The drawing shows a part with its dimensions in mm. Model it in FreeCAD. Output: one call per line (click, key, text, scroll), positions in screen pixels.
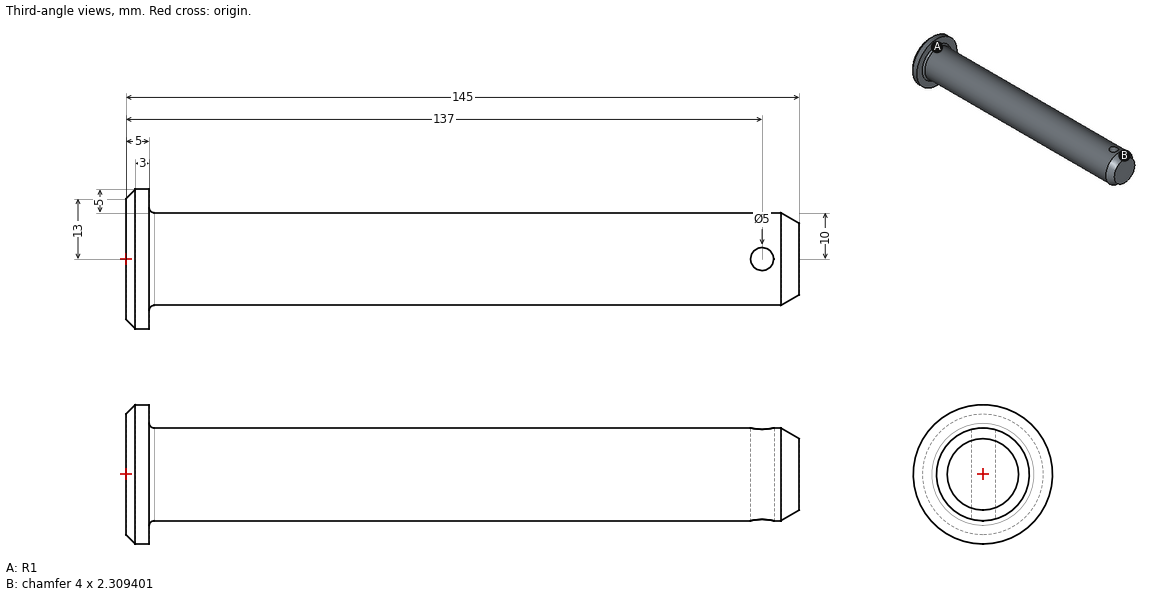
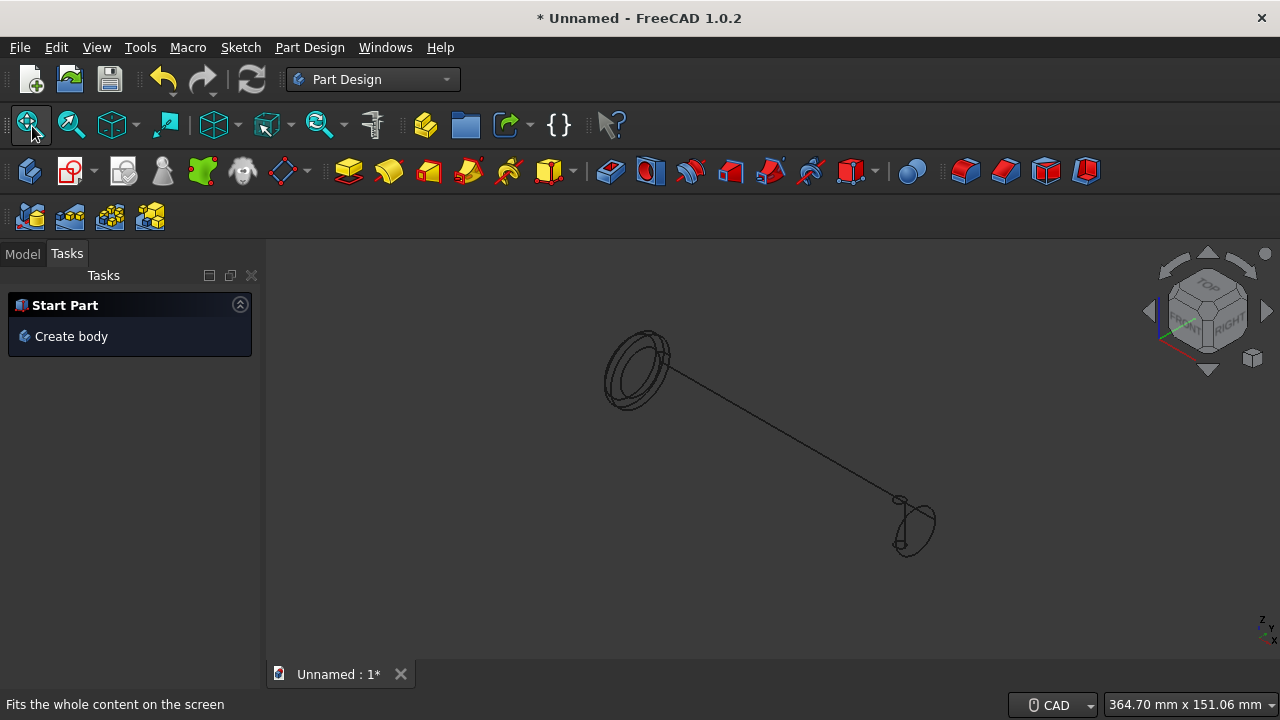
click(621, 383)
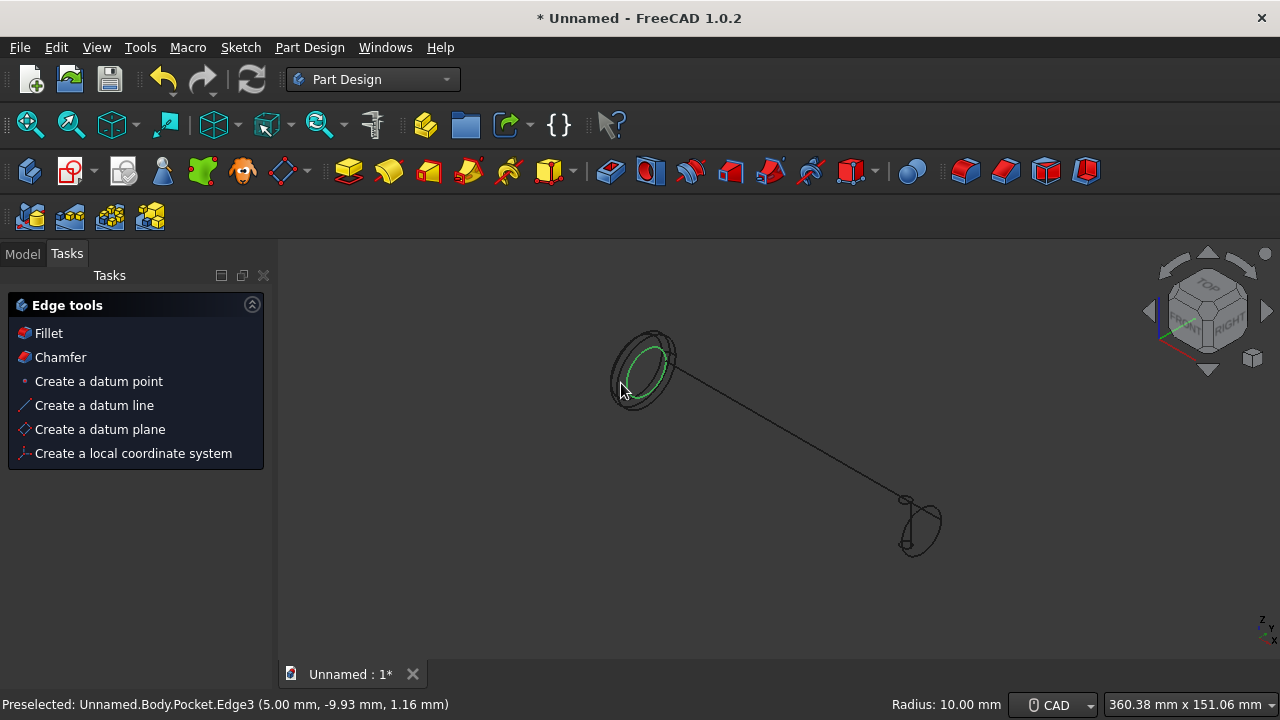
key(v)
key(1)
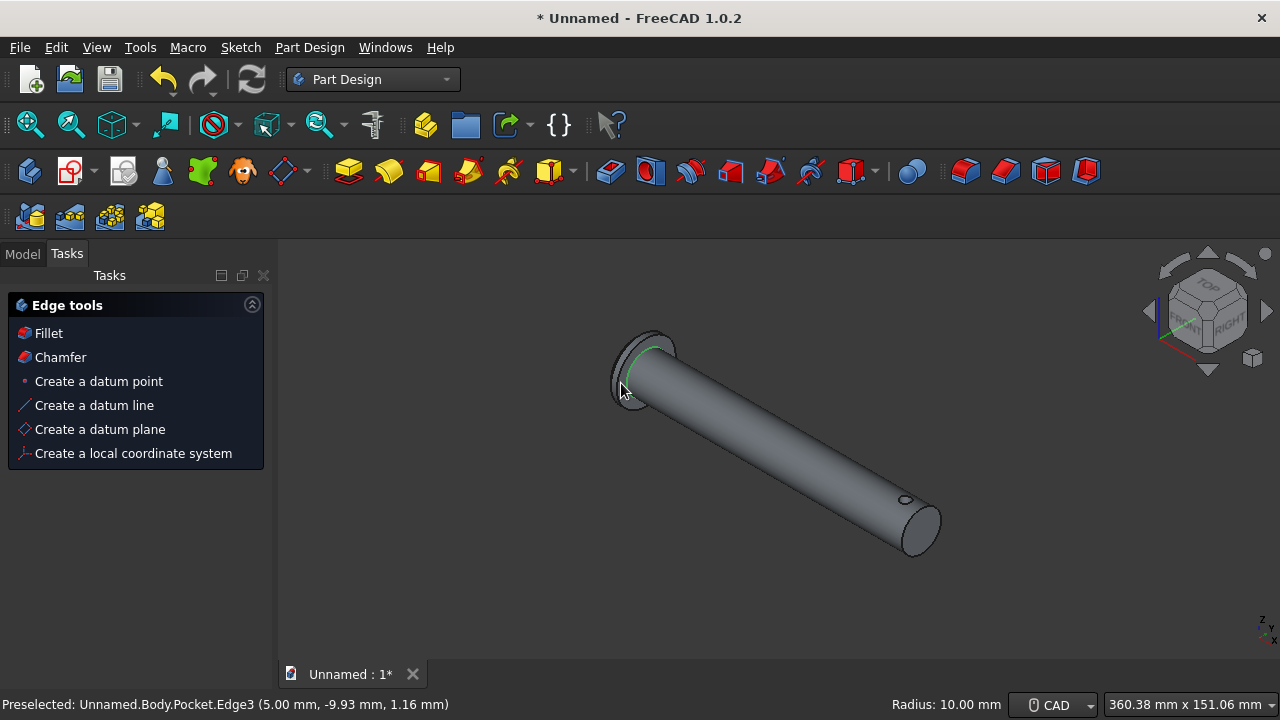
click(966, 172)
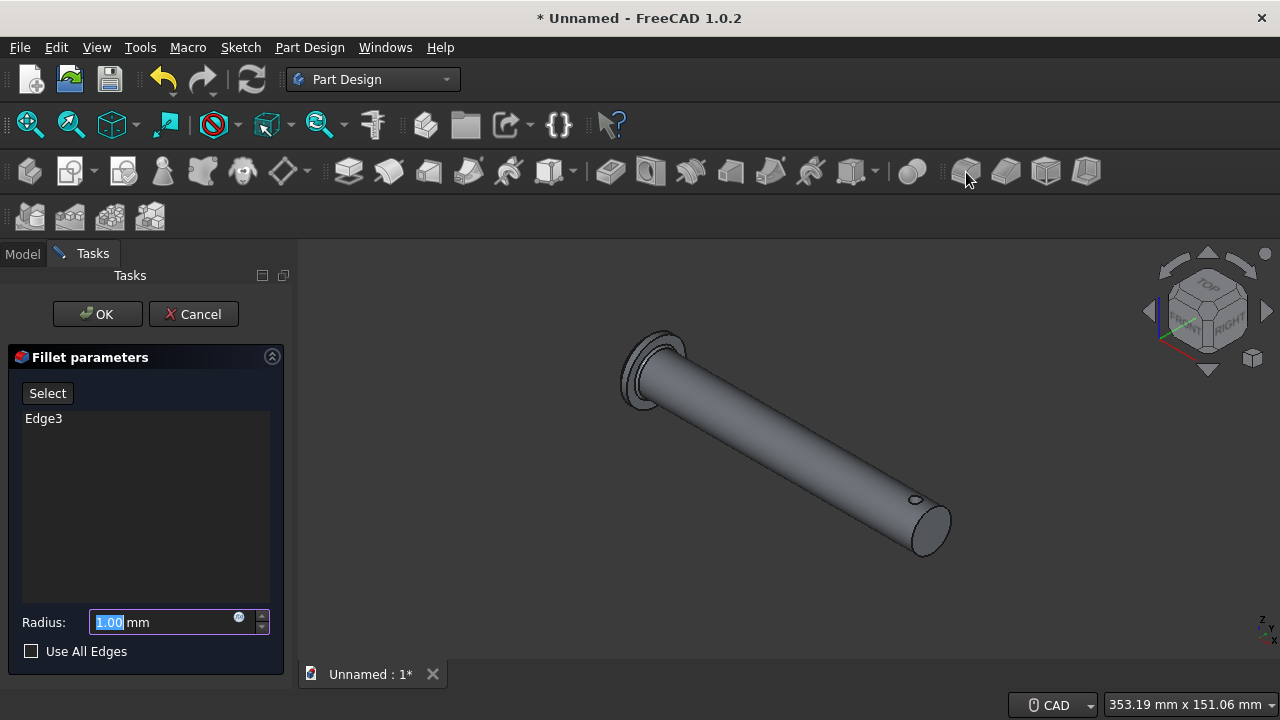
text(1)
key(Tab)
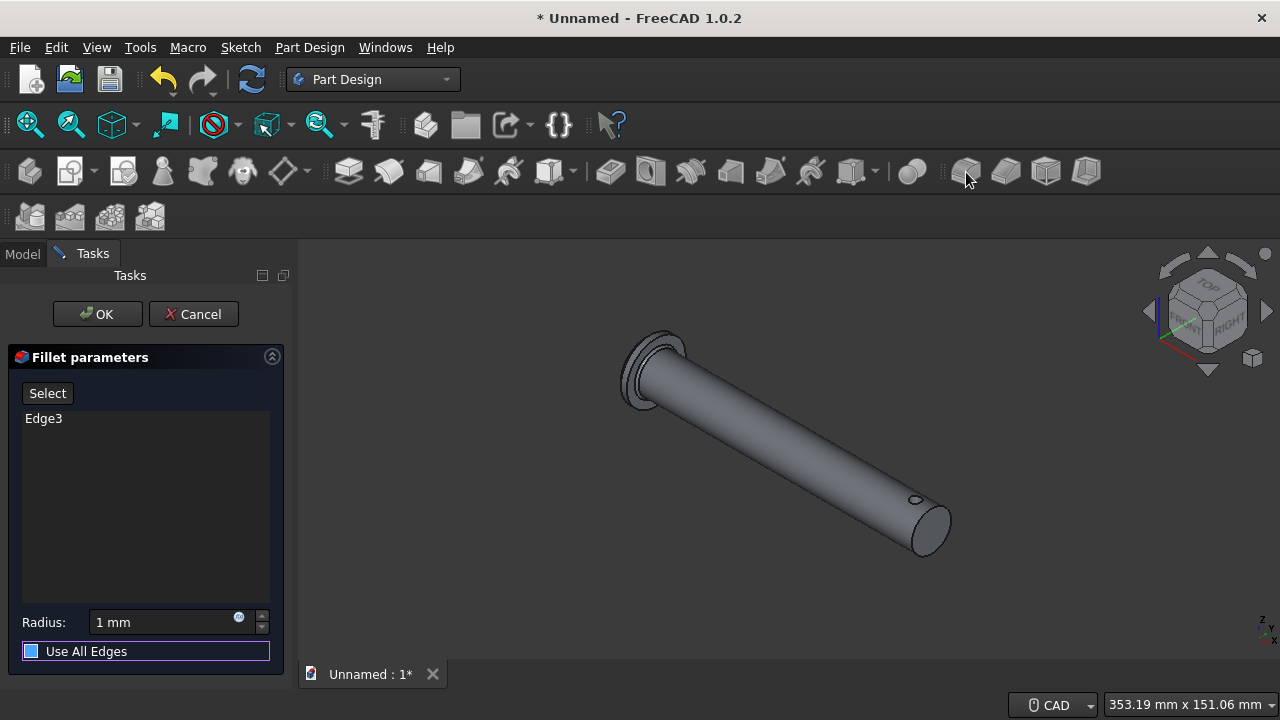
click(98, 314)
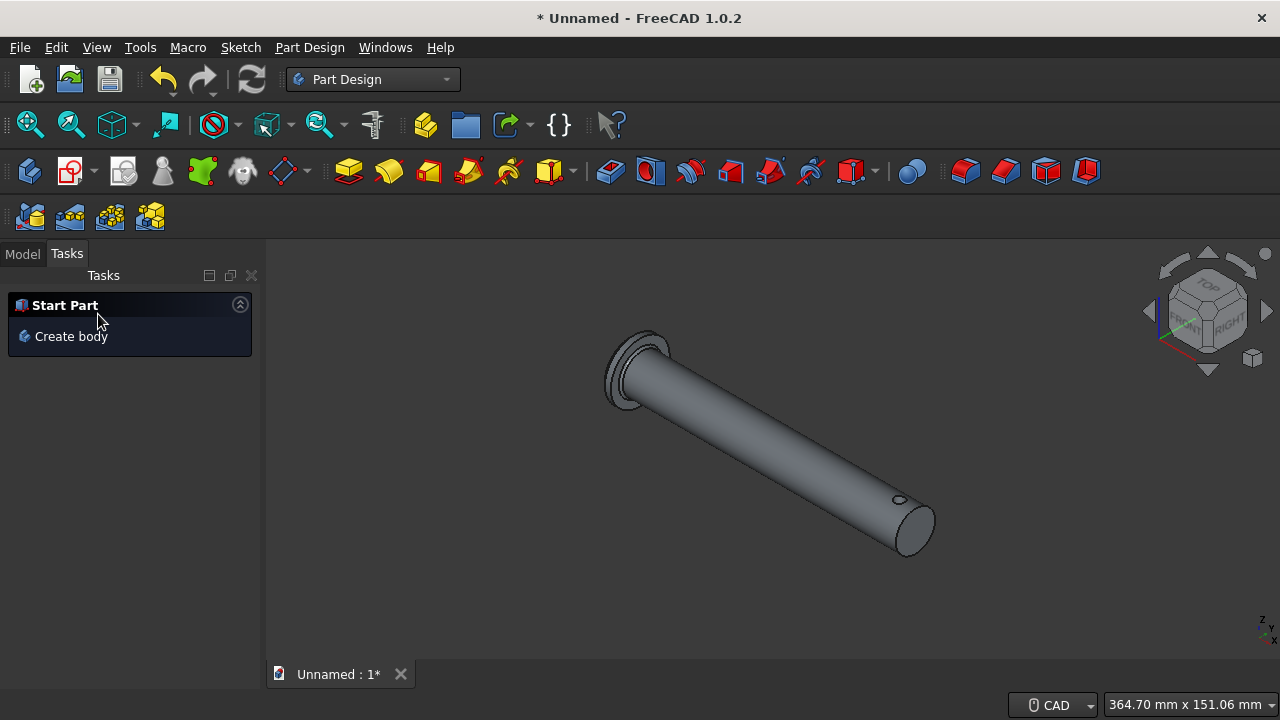
click(896, 542)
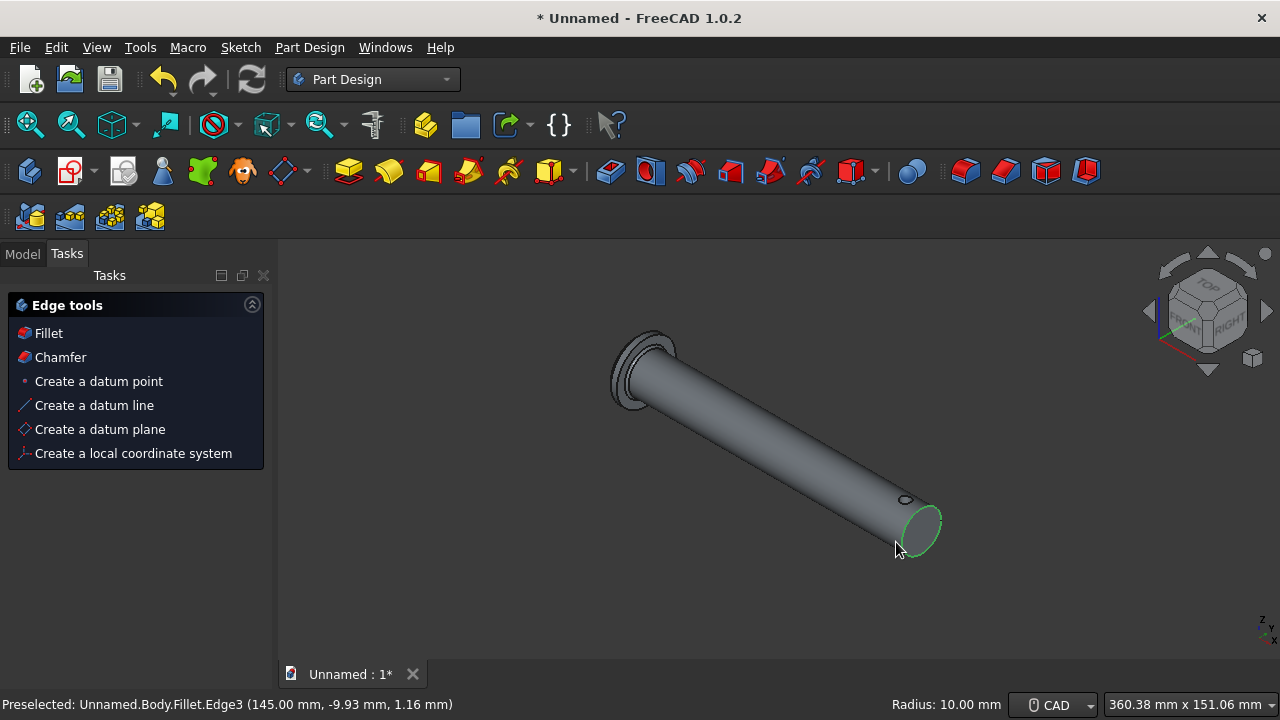
click(1006, 172)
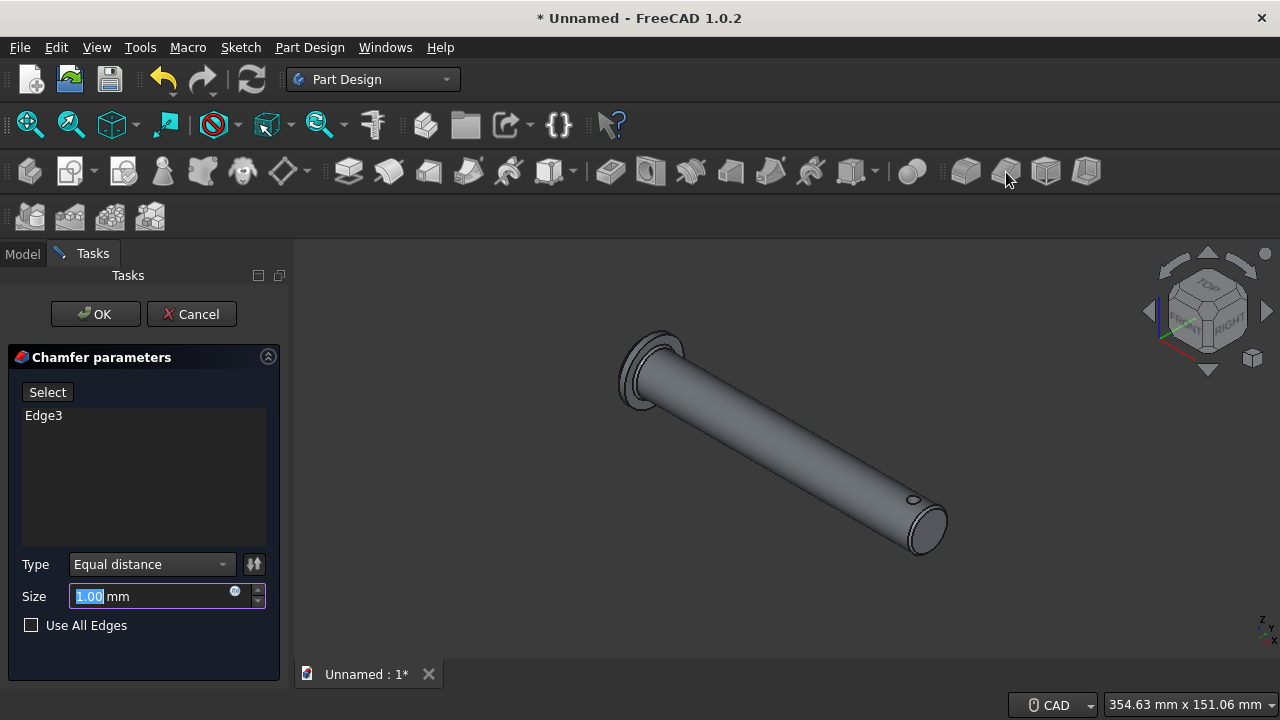
text(4)
key(Tab)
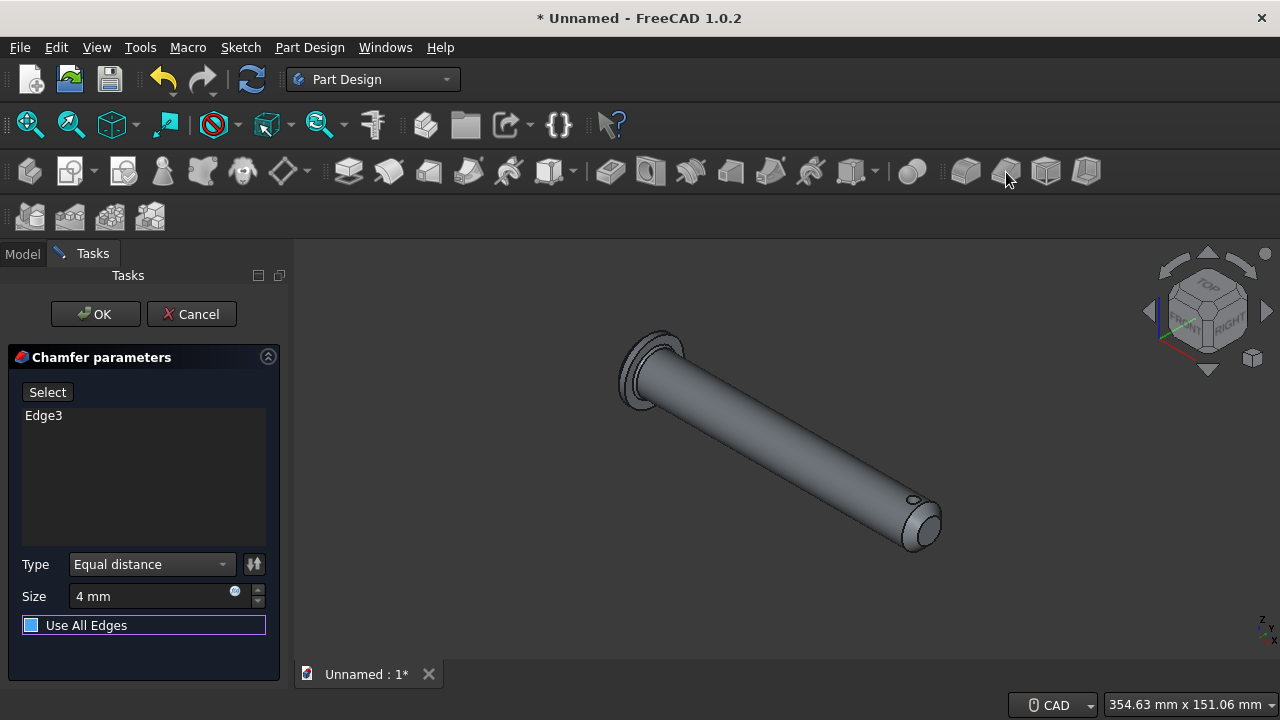
click(153, 564)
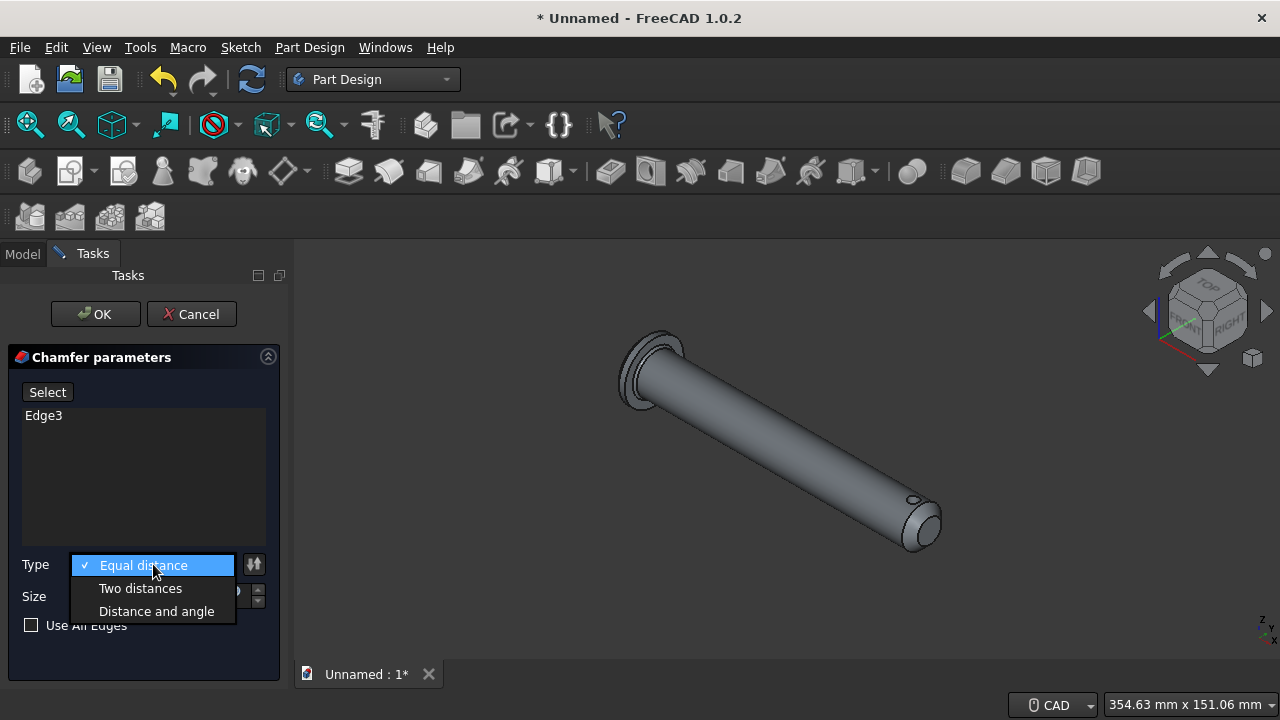
click(152, 588)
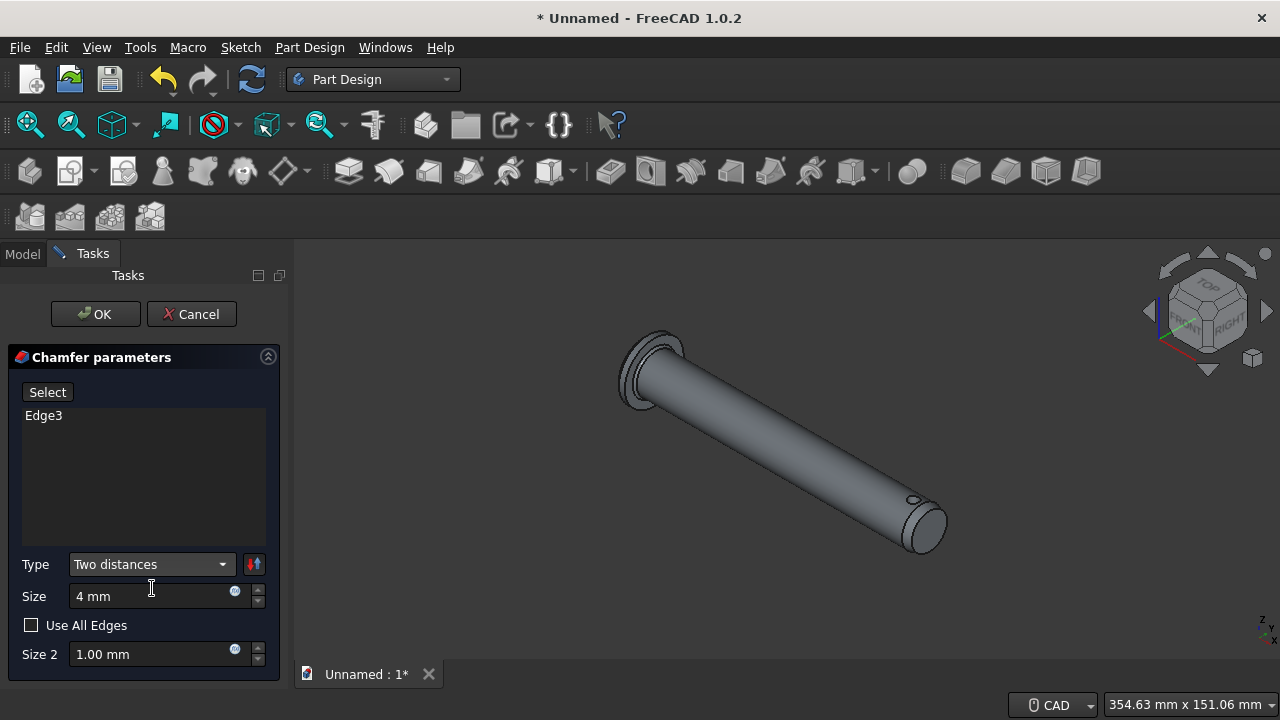
triple_click(160, 654)